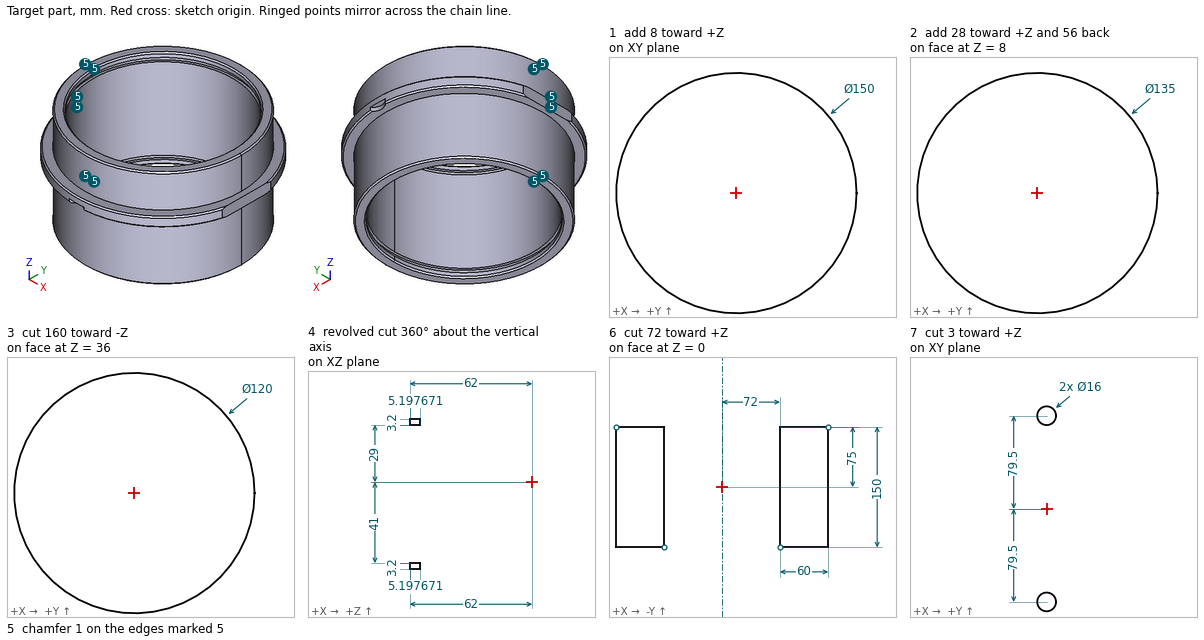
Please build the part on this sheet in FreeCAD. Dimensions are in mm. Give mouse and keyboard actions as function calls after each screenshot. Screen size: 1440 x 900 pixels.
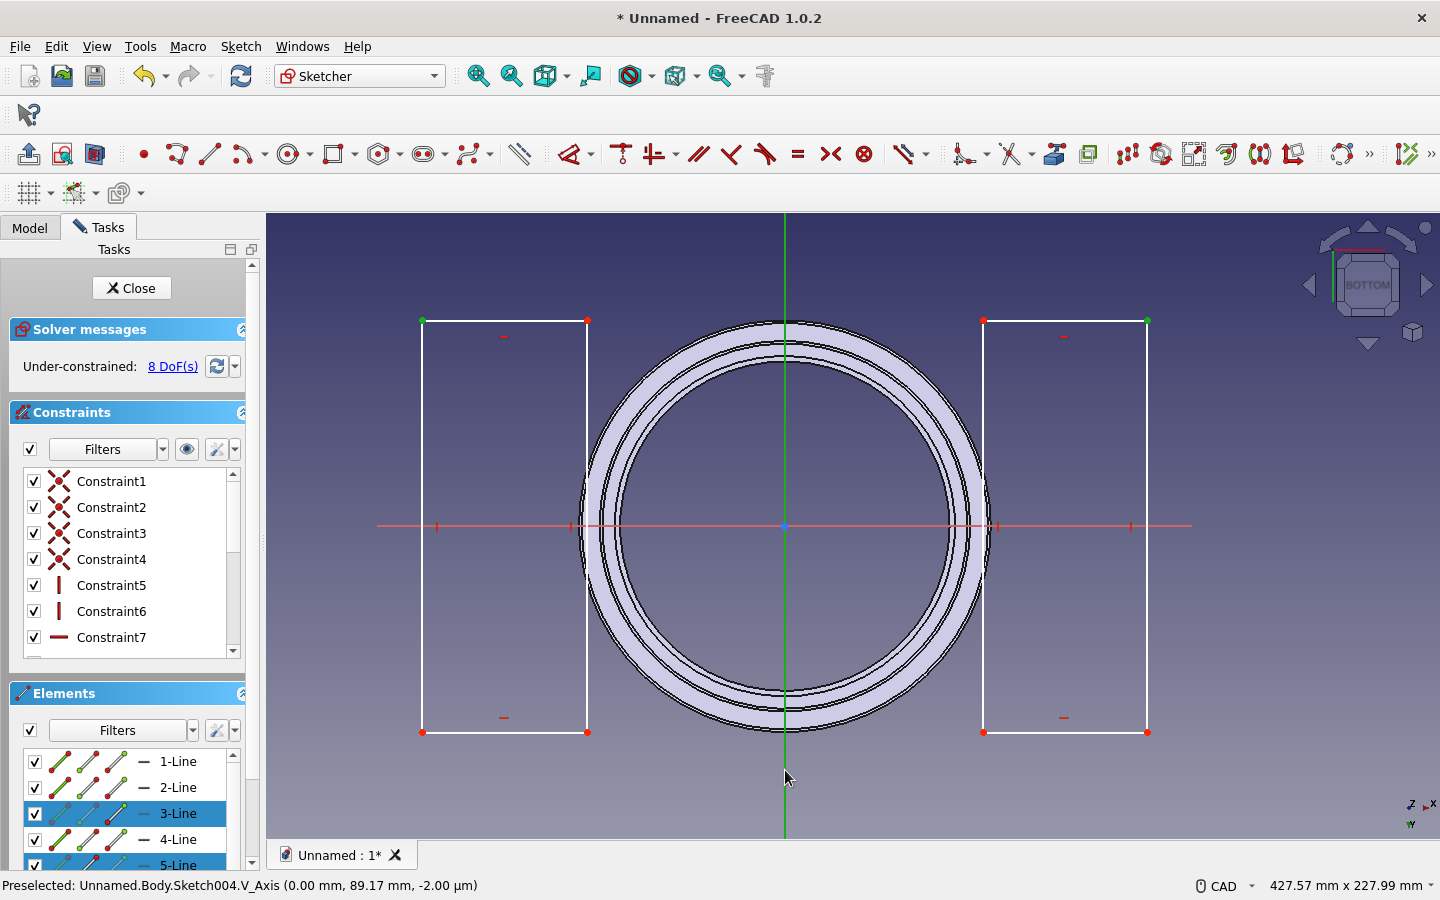
key(s)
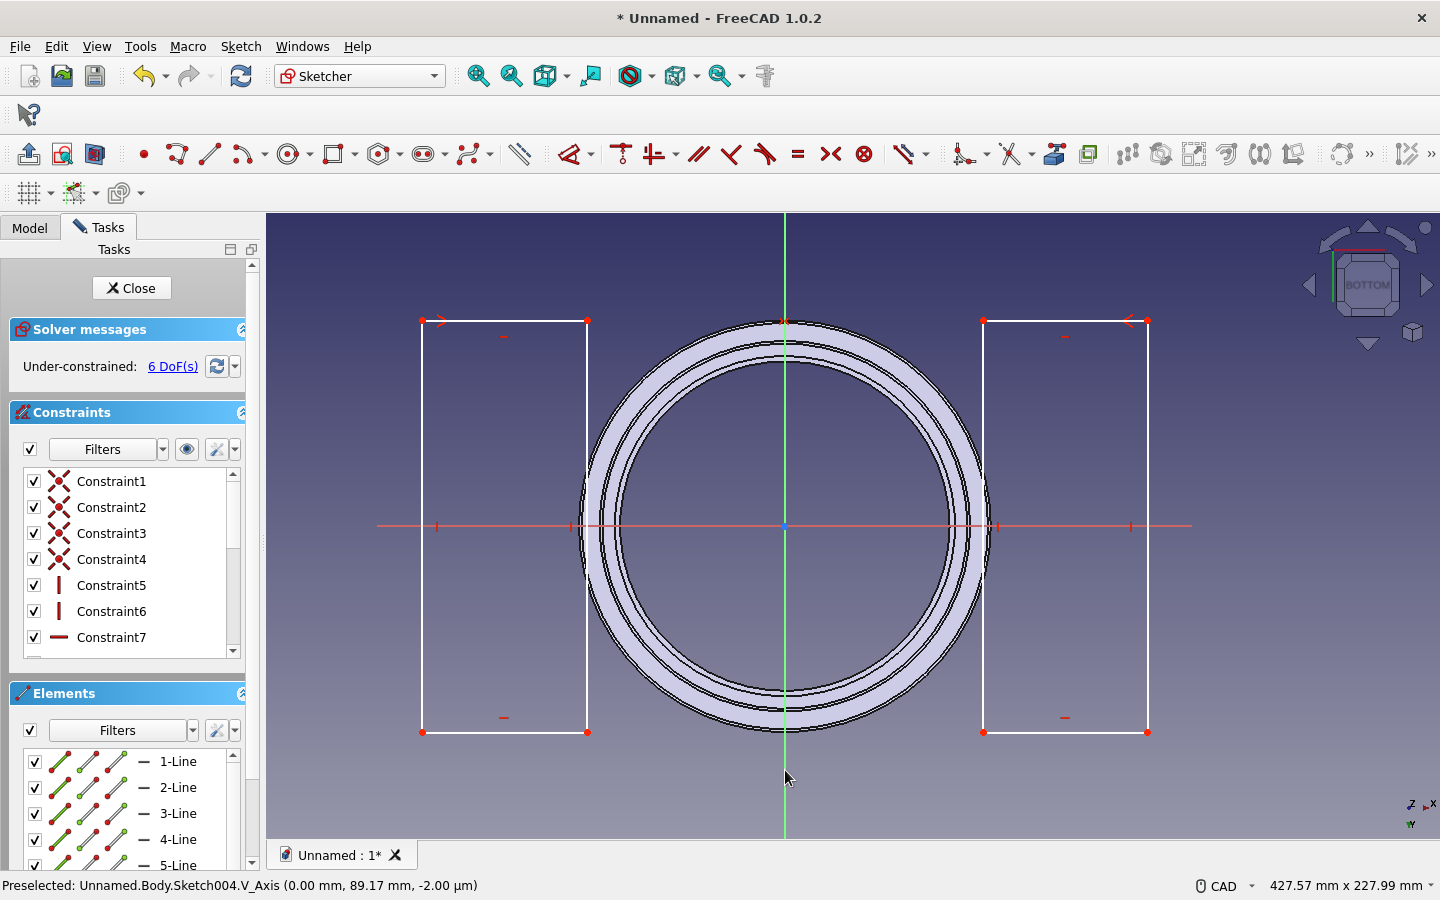
click(983, 733)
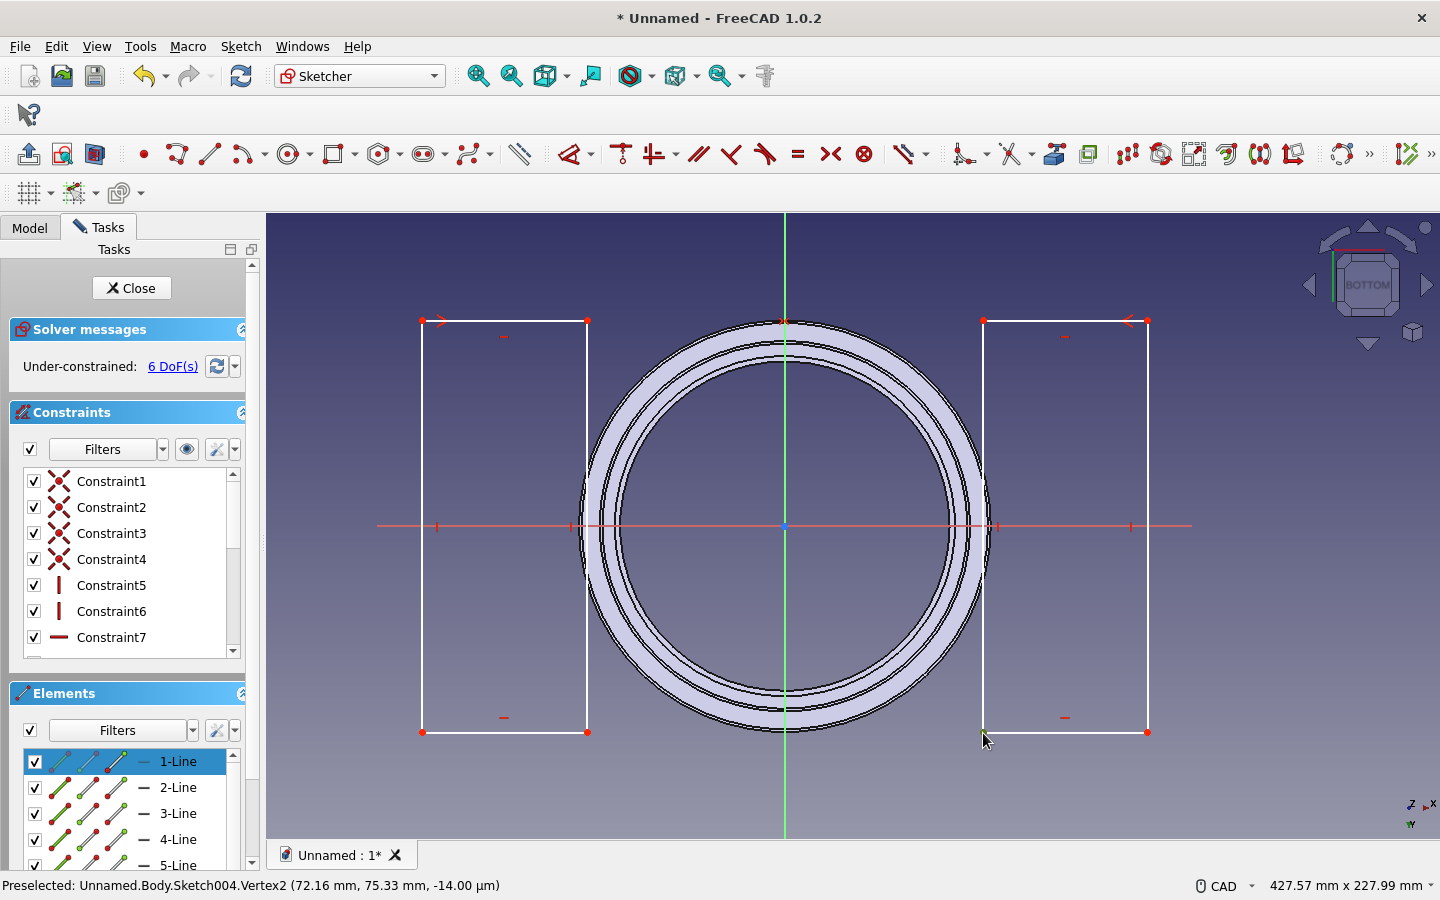
click(587, 733)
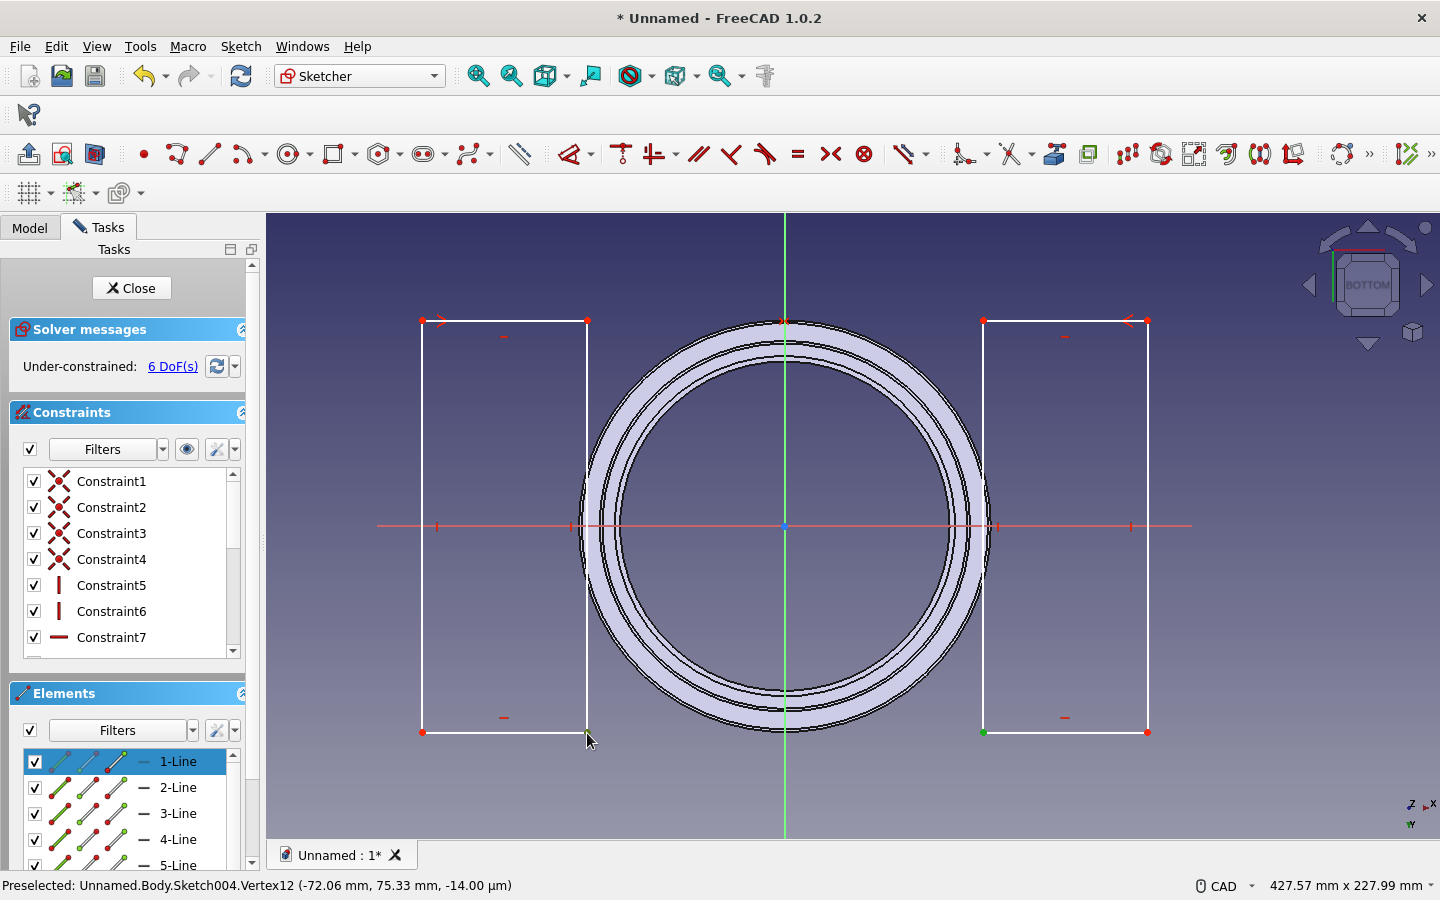
click(785, 770)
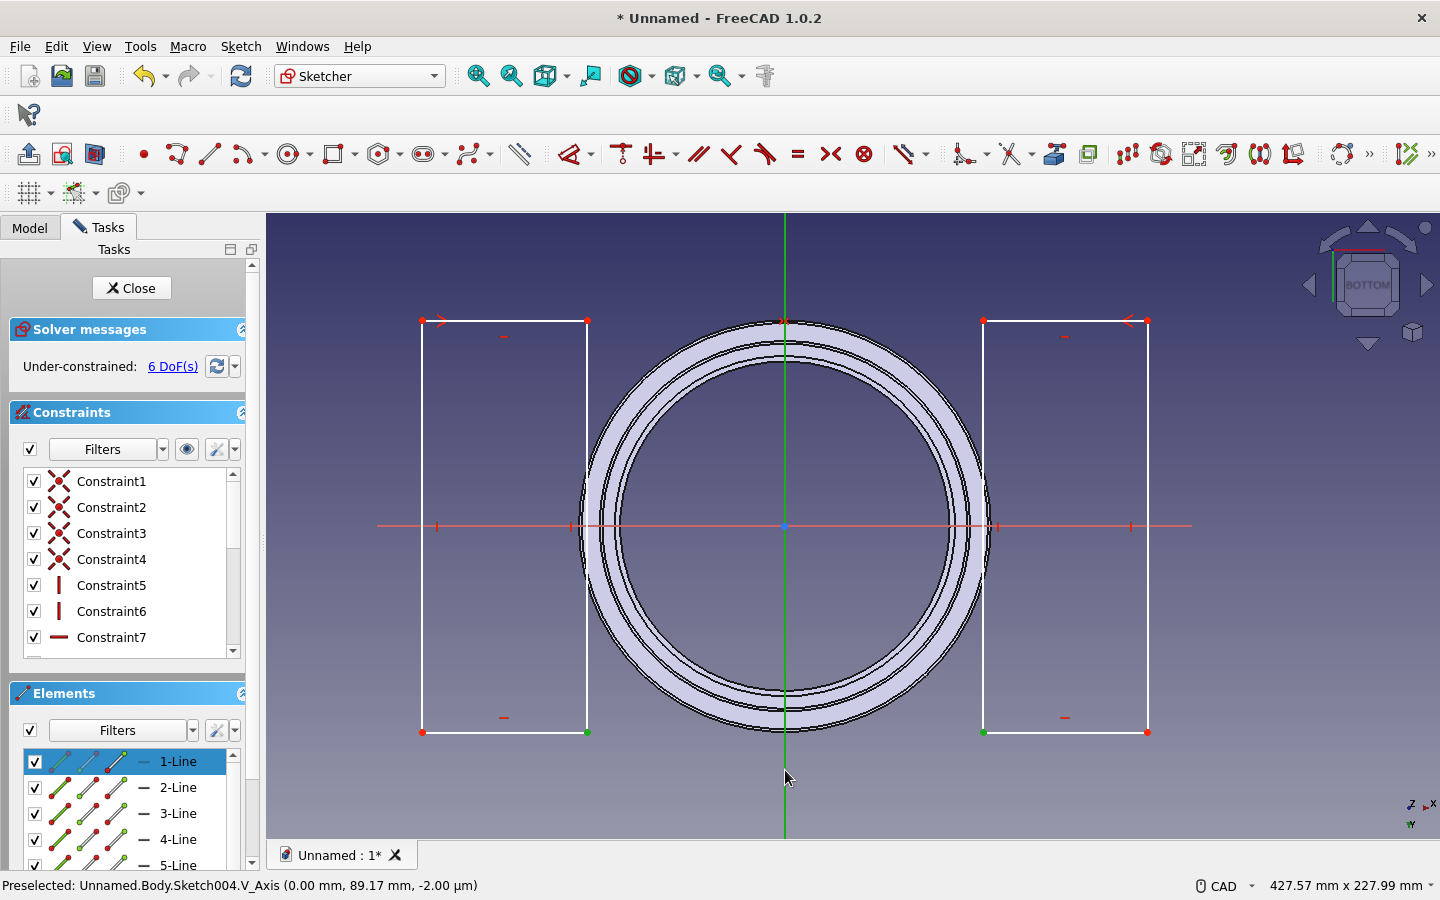
key(s)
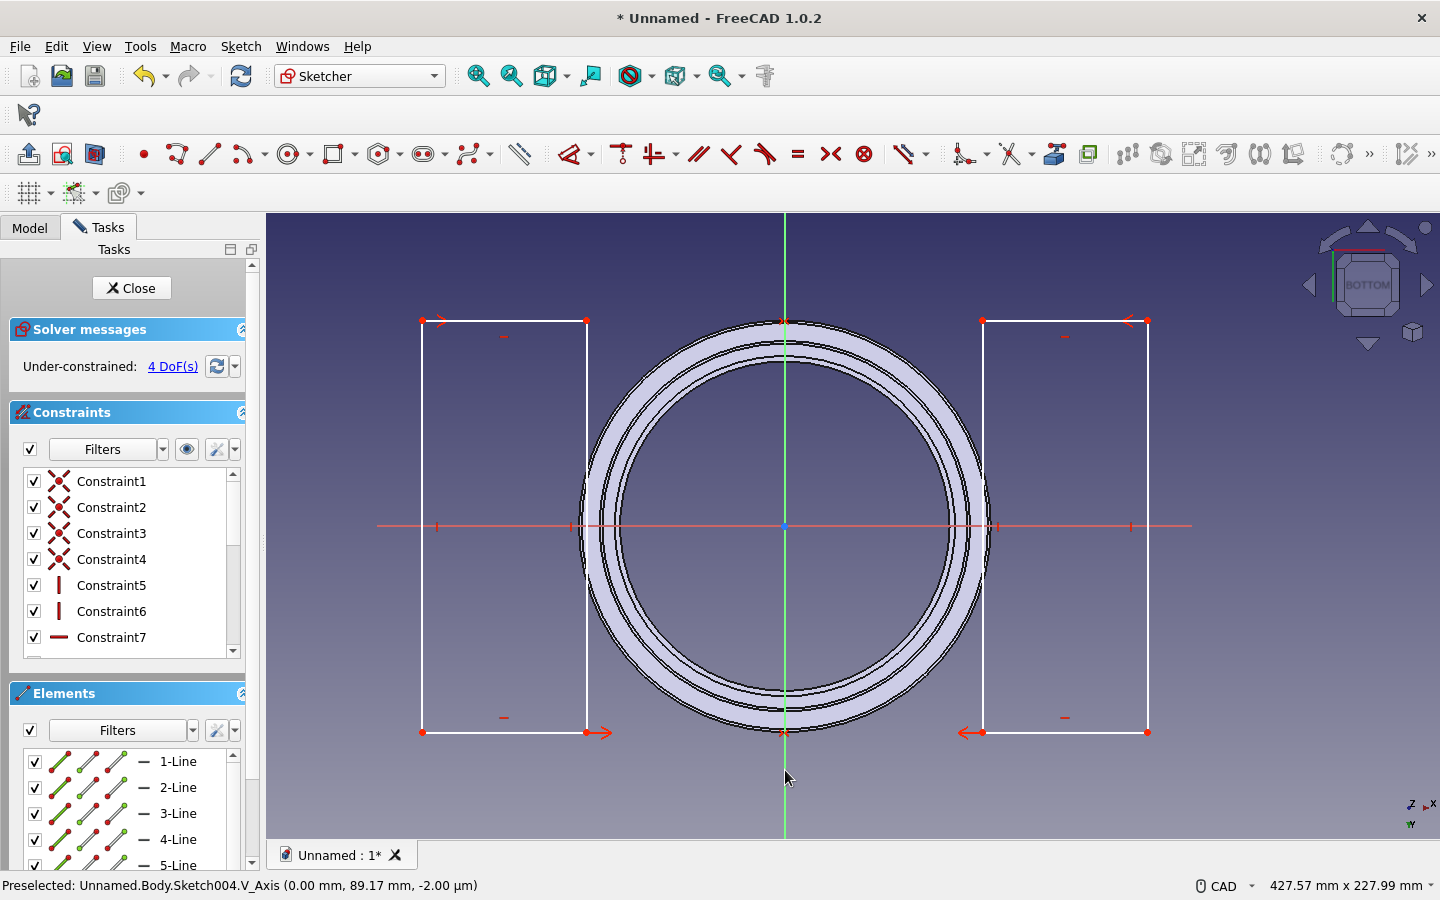
key(d)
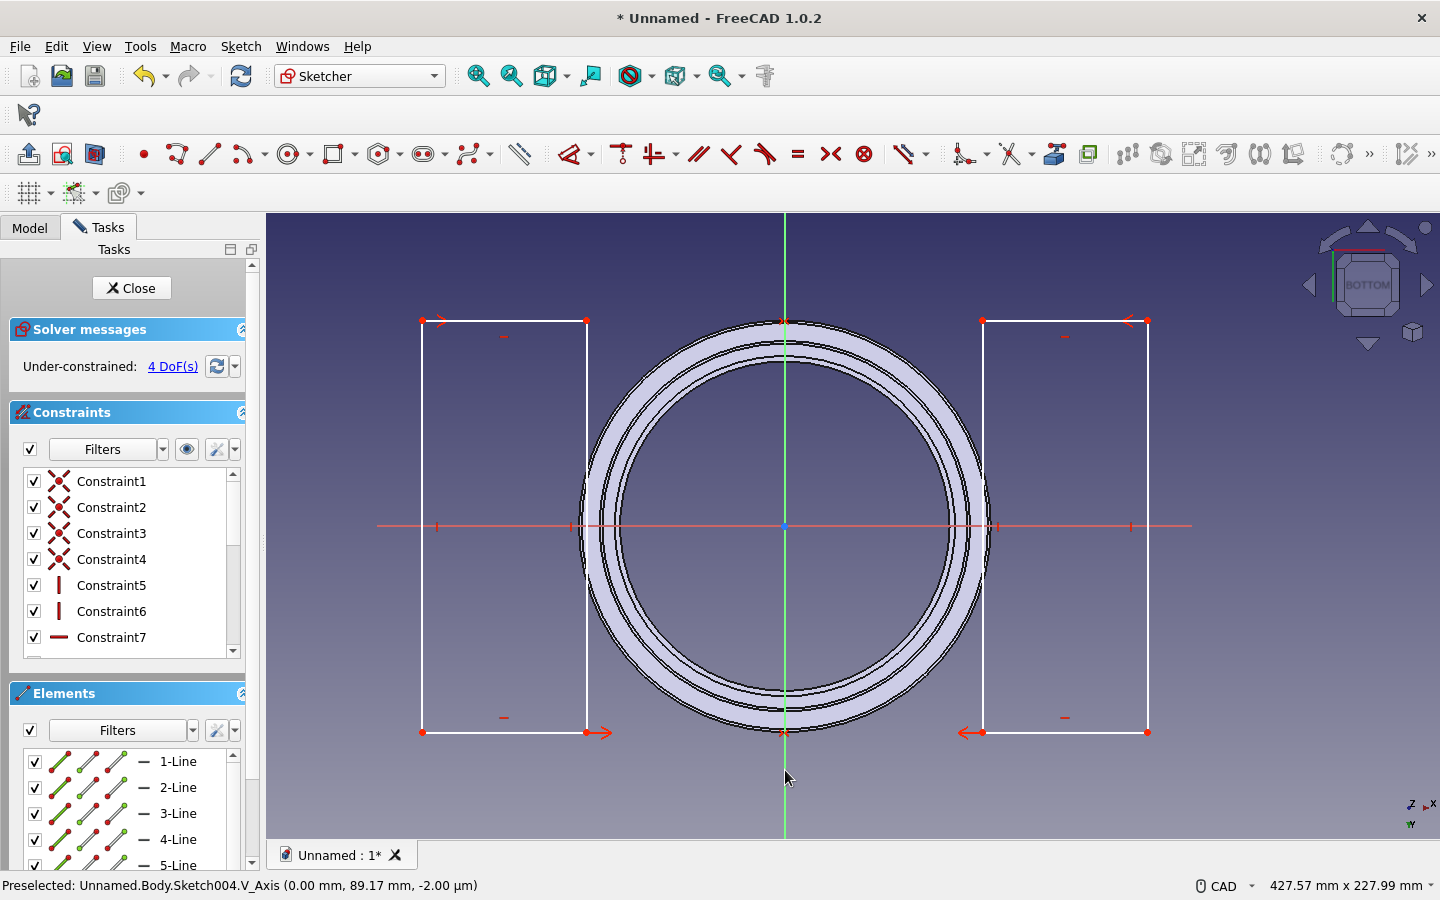
click(1032, 733)
click(1065, 767)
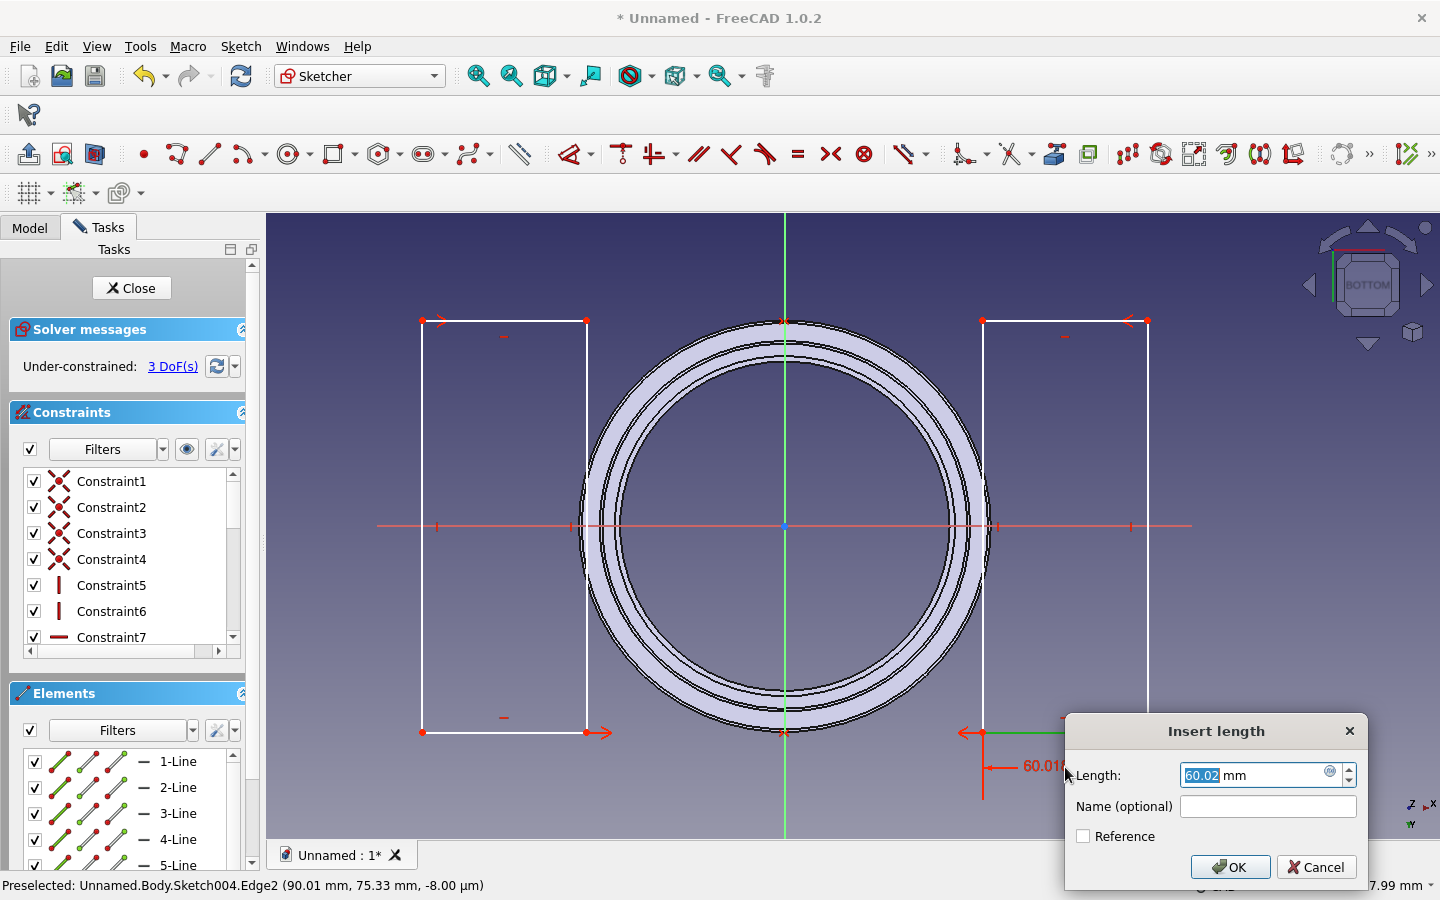
text(60)
key(Return)